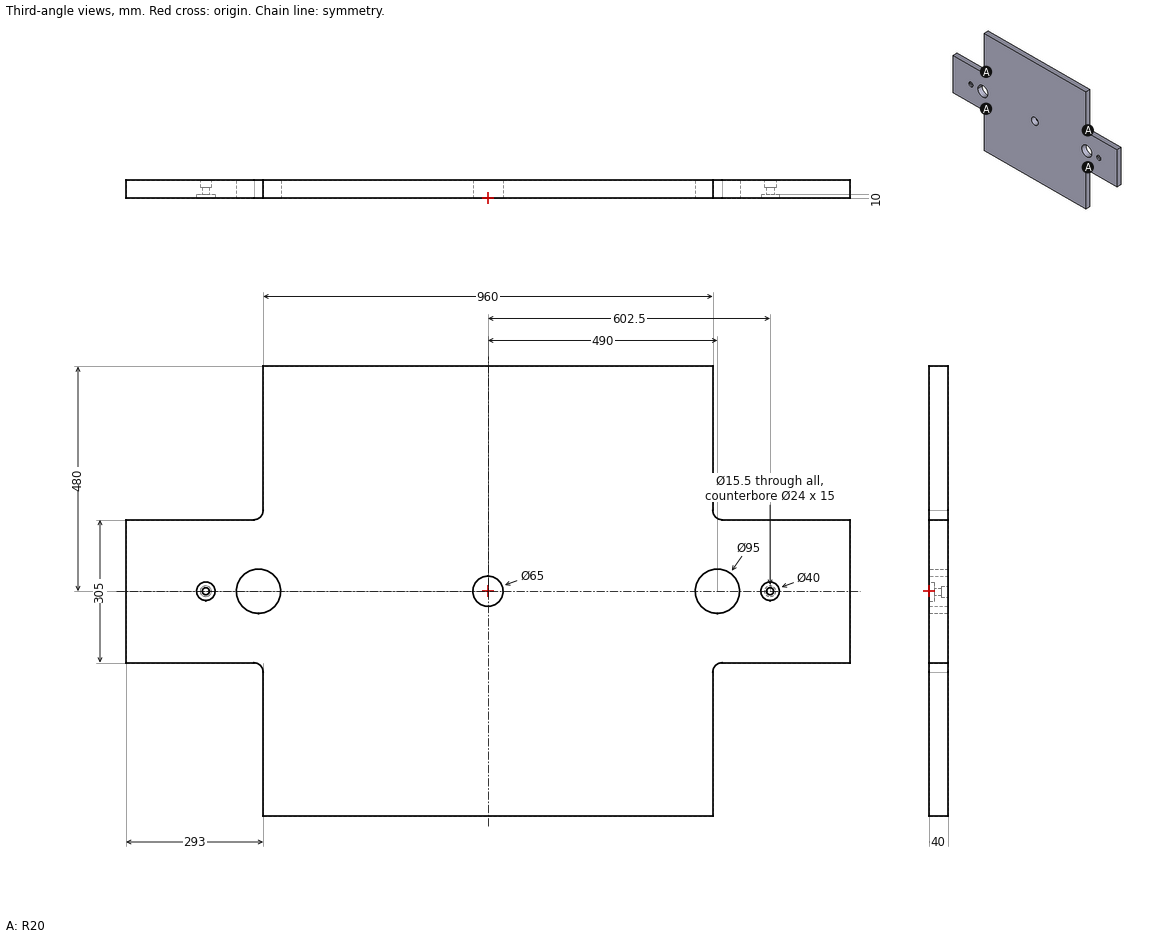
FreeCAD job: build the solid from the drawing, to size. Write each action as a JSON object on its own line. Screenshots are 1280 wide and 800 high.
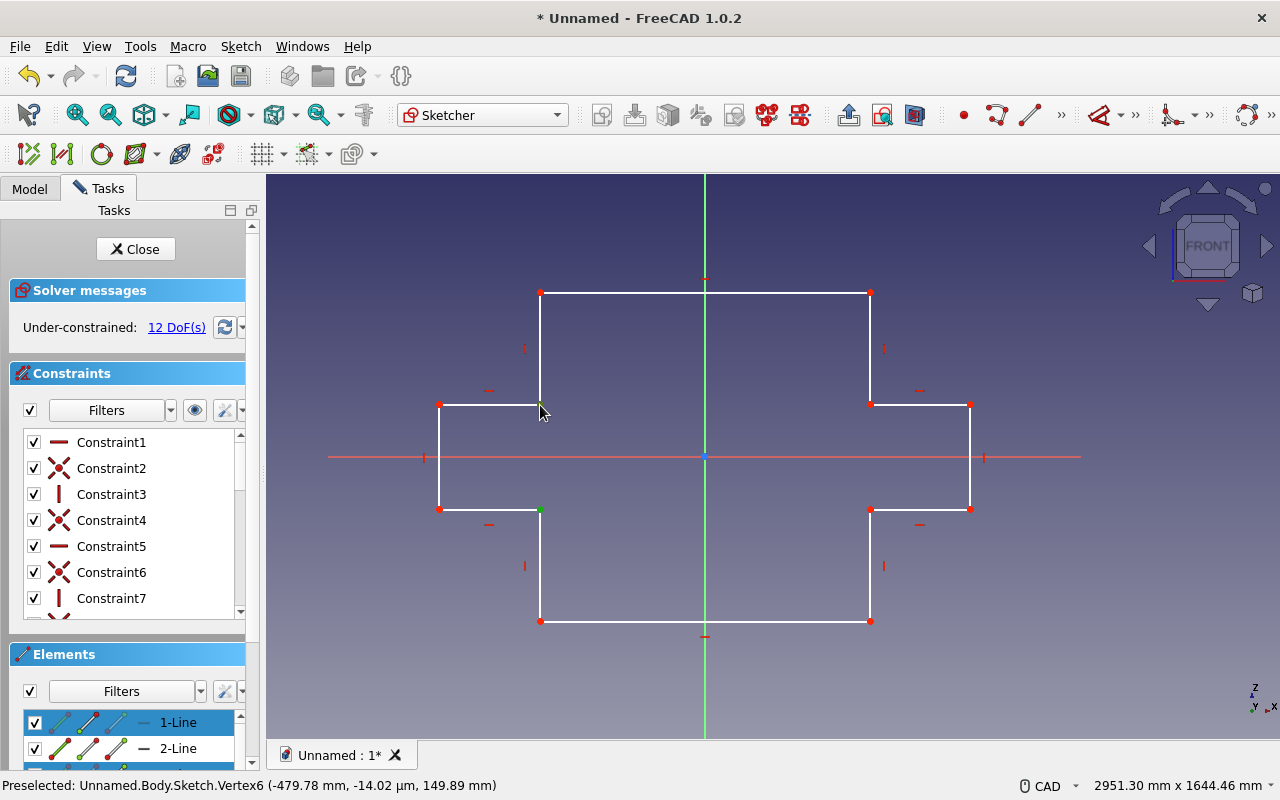
{"action": "left_click", "coordinate": [353, 456]}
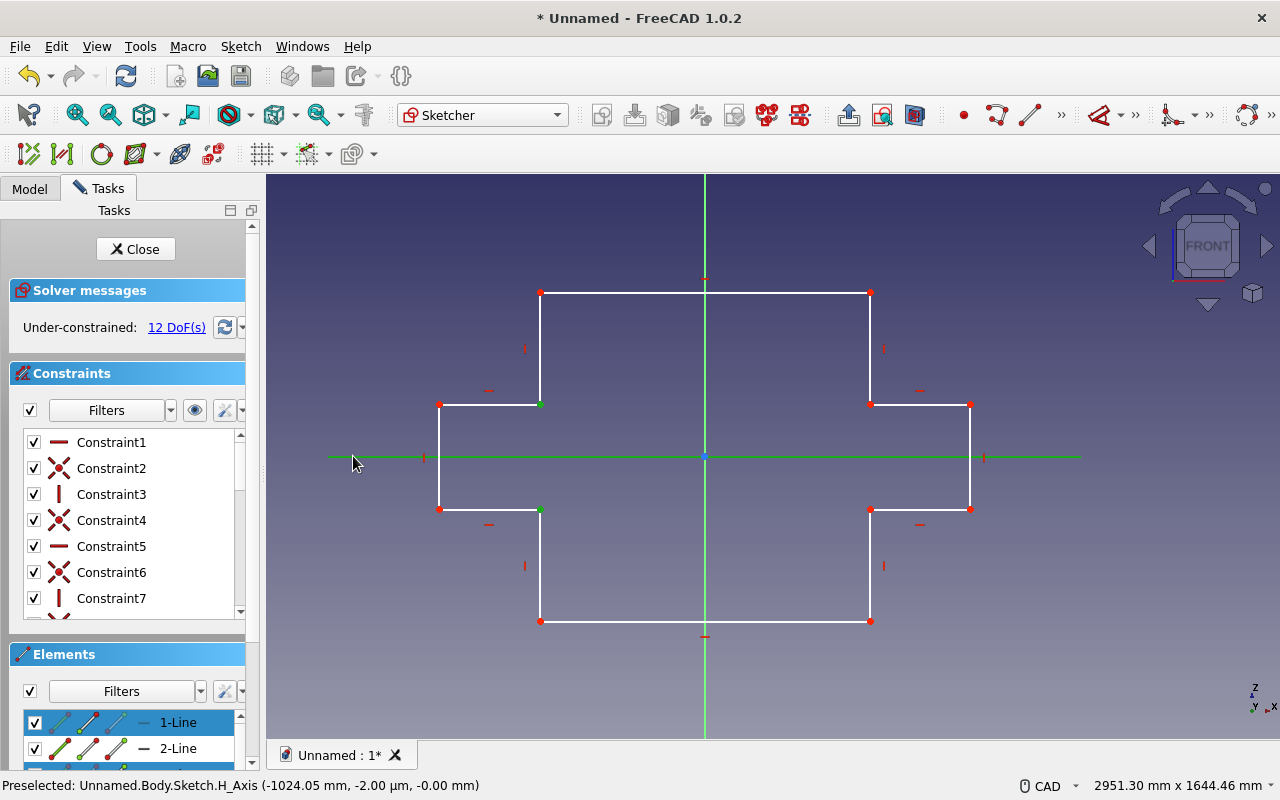
{"action": "key", "text": "s"}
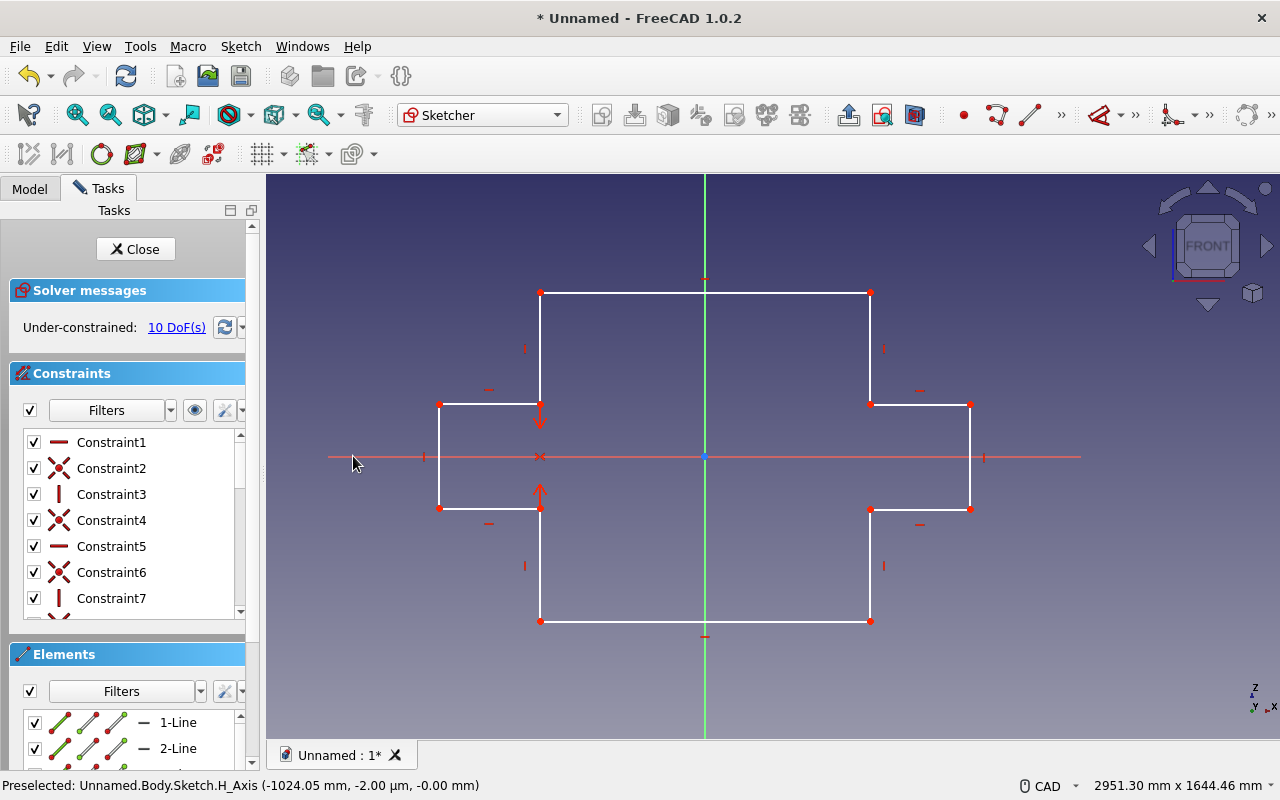
{"action": "left_click", "coordinate": [540, 404]}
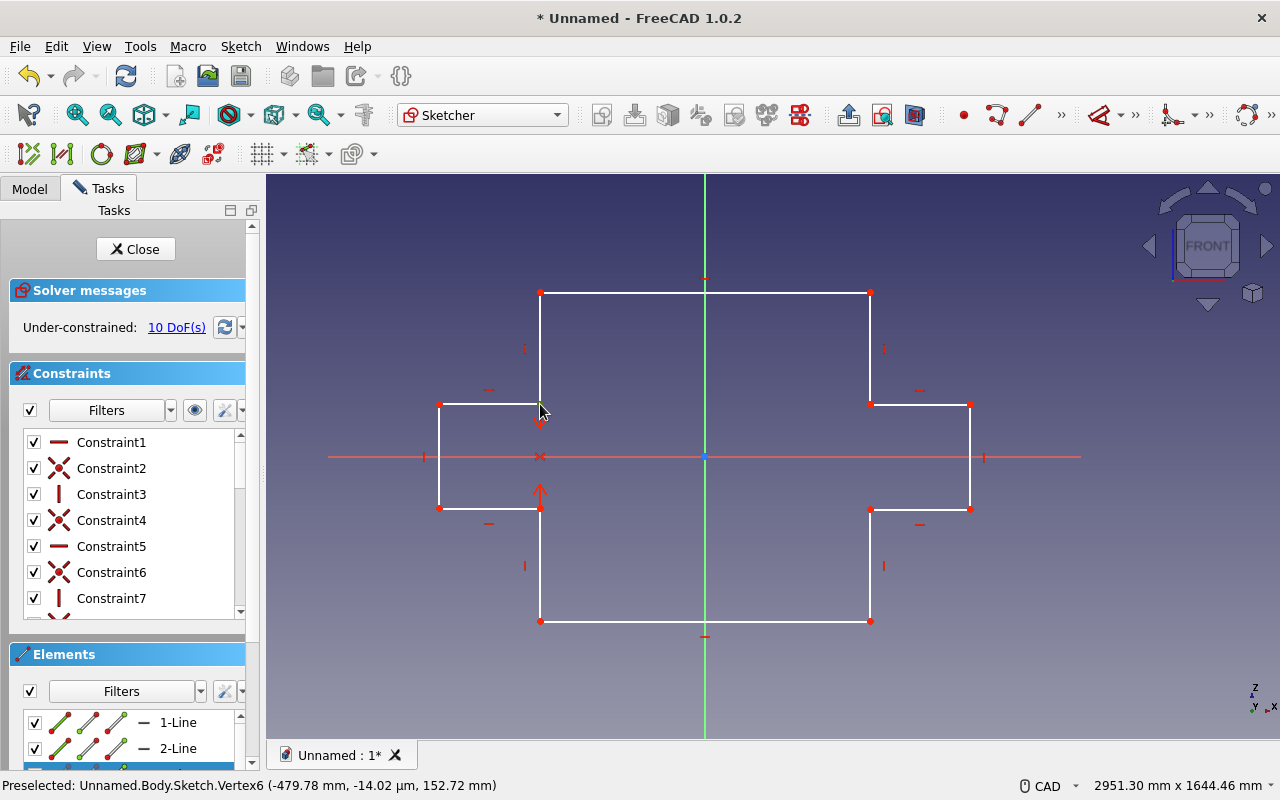
{"action": "left_click", "coordinate": [870, 405]}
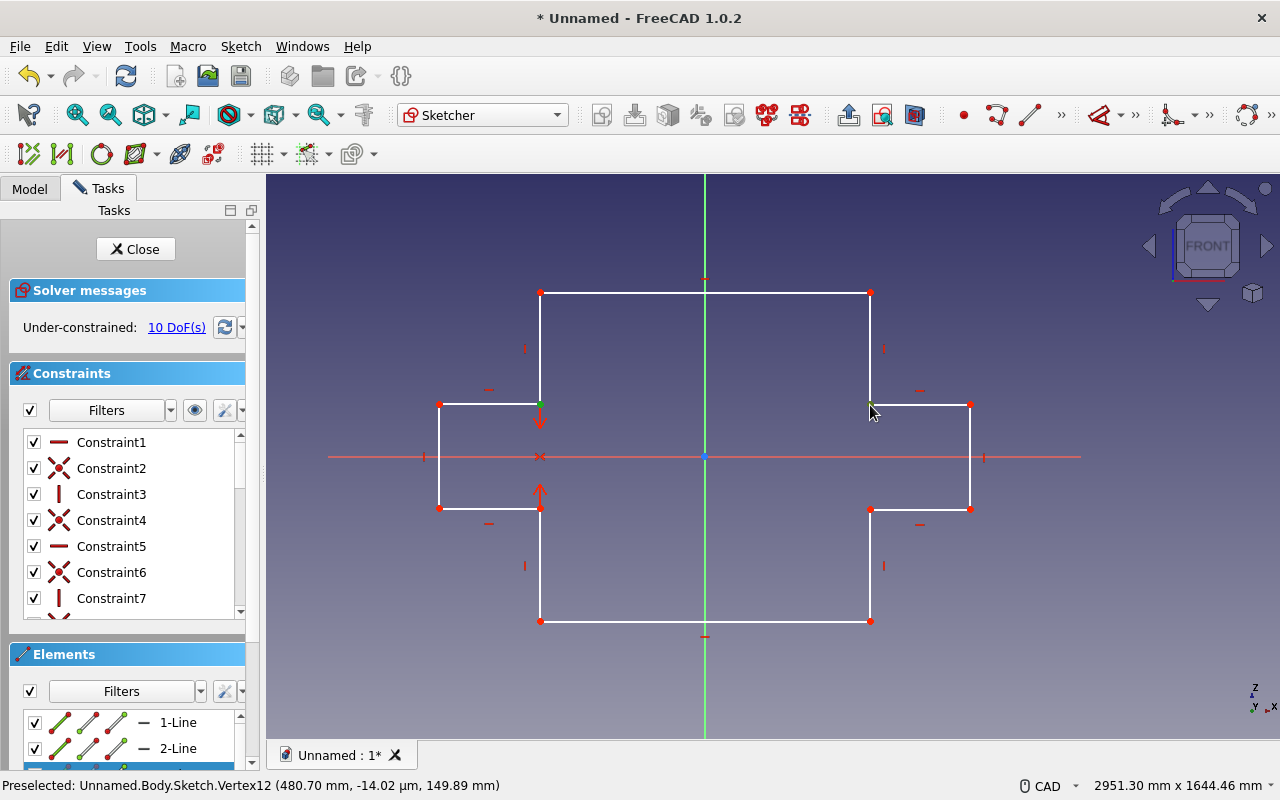
{"action": "left_click", "coordinate": [705, 675]}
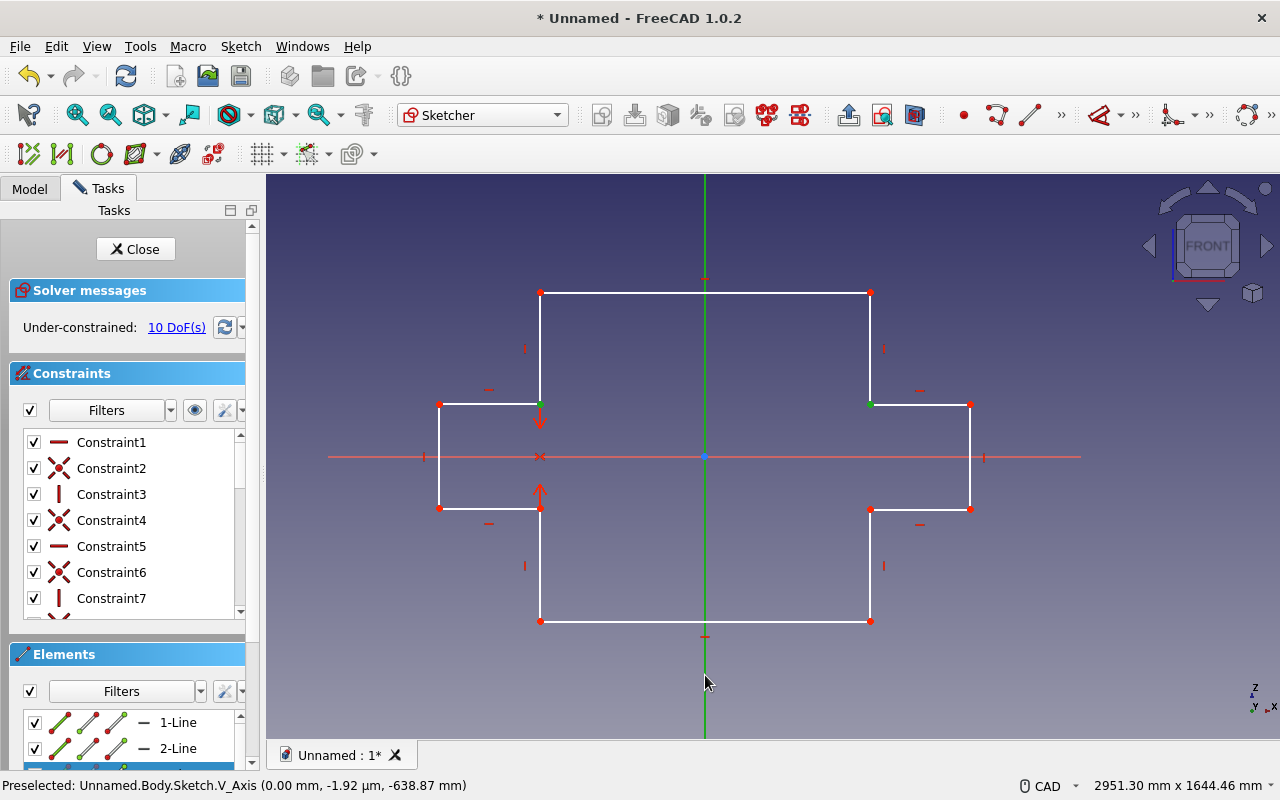
{"action": "key", "text": "s"}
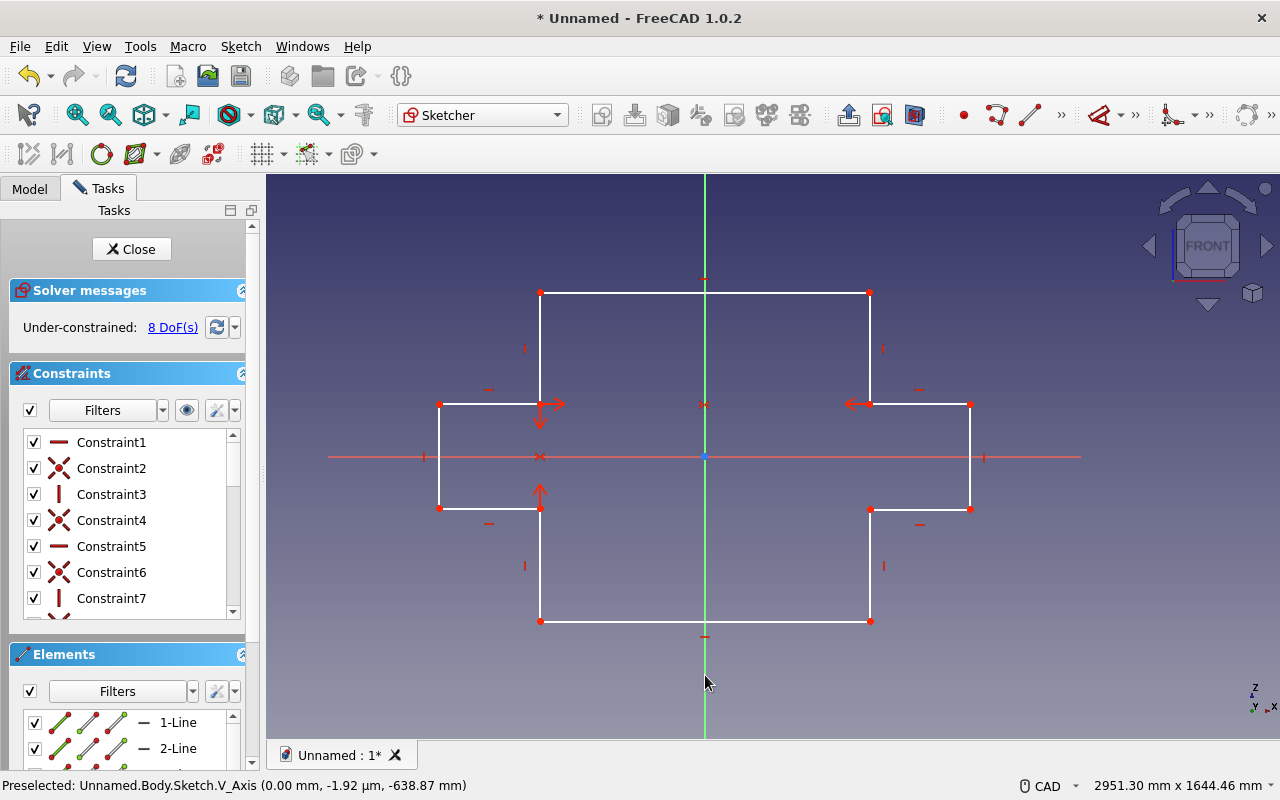
{"action": "left_click", "coordinate": [439, 509]}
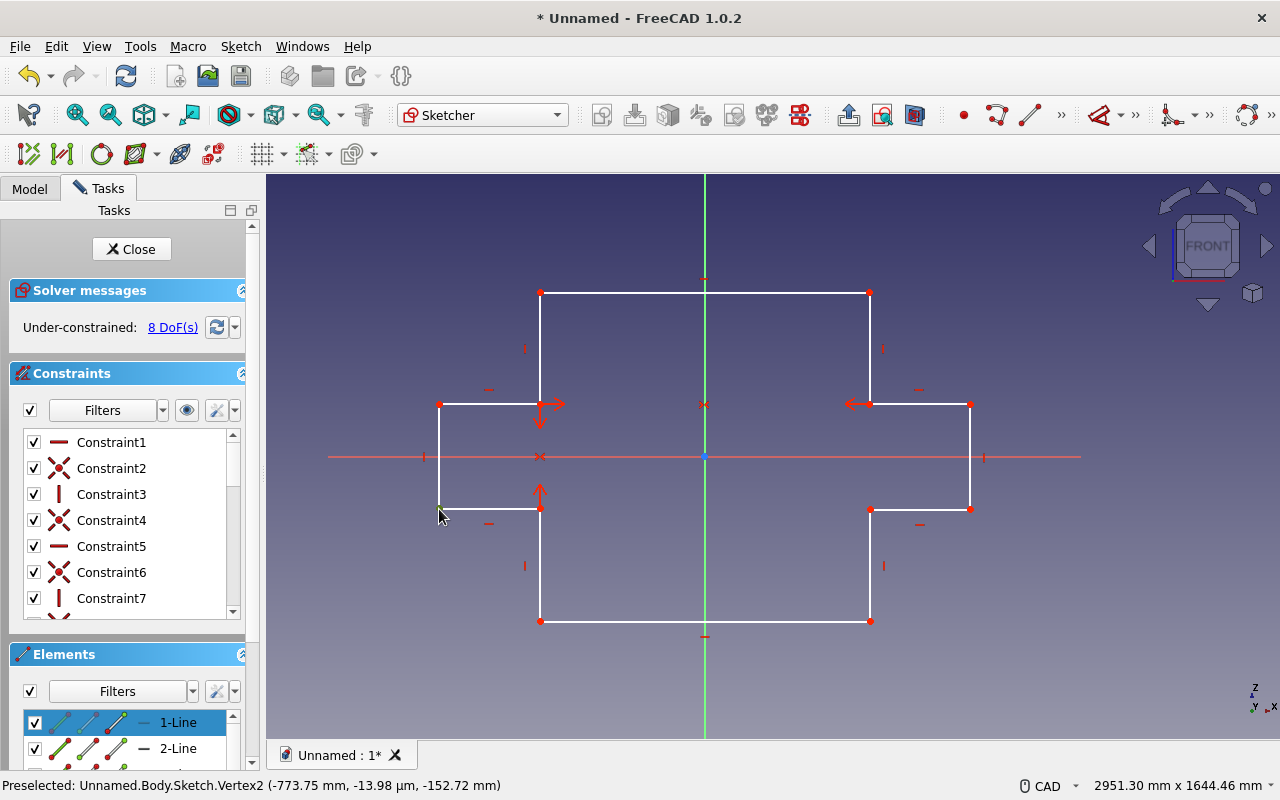
{"action": "left_click", "coordinate": [970, 510]}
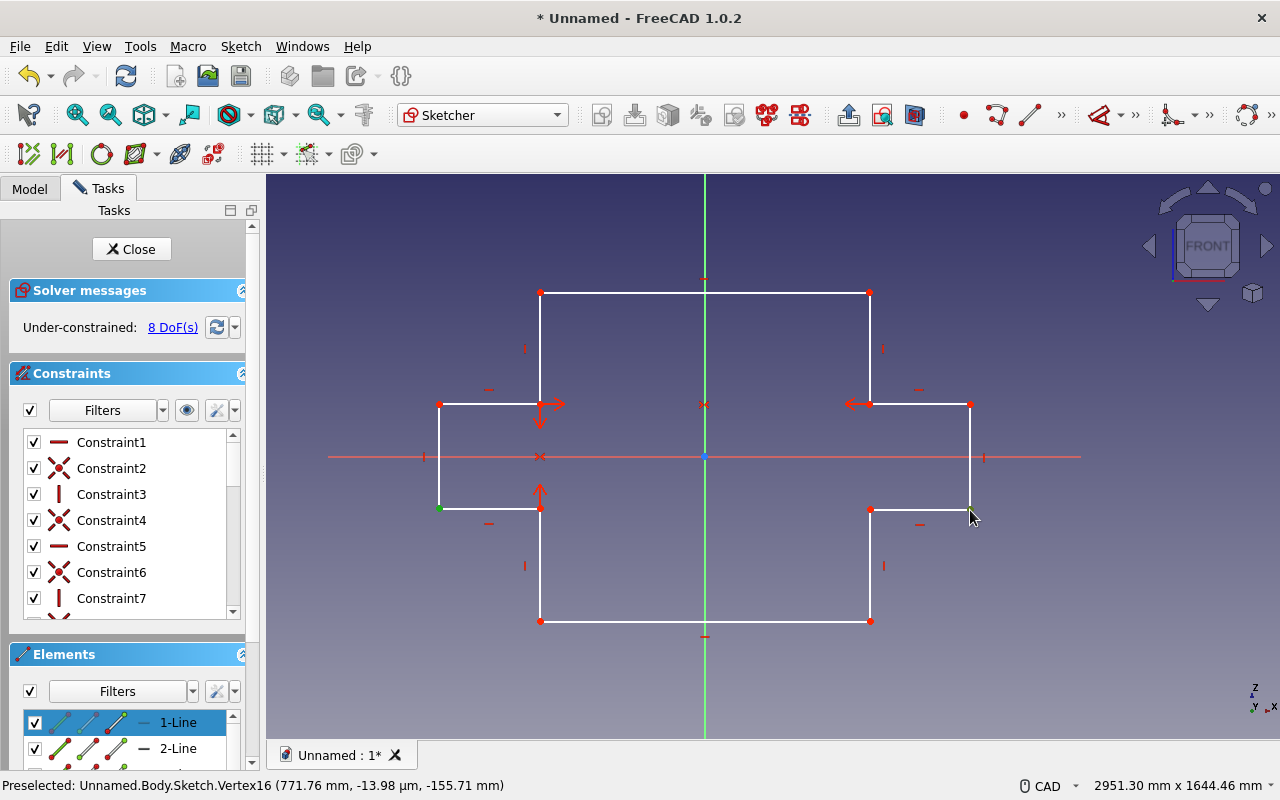
{"action": "left_click", "coordinate": [705, 675]}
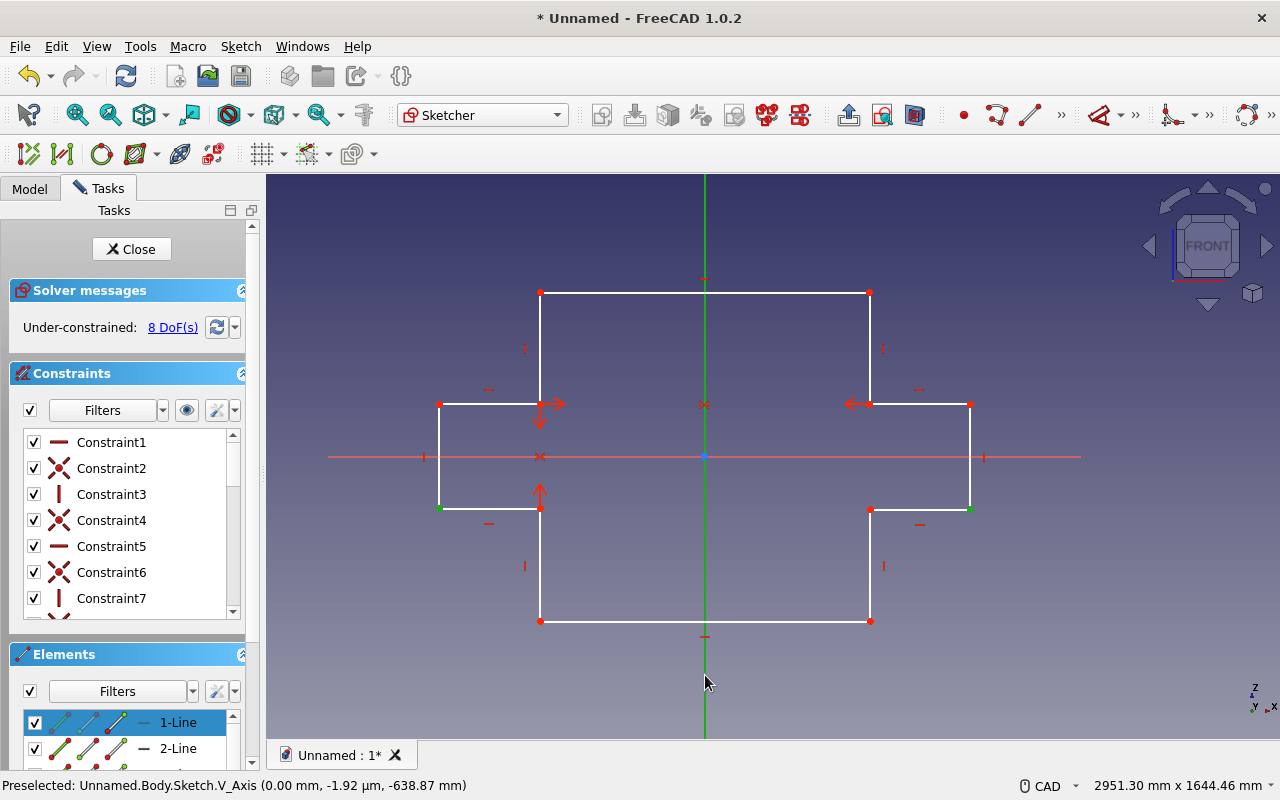
{"action": "key", "text": "s"}